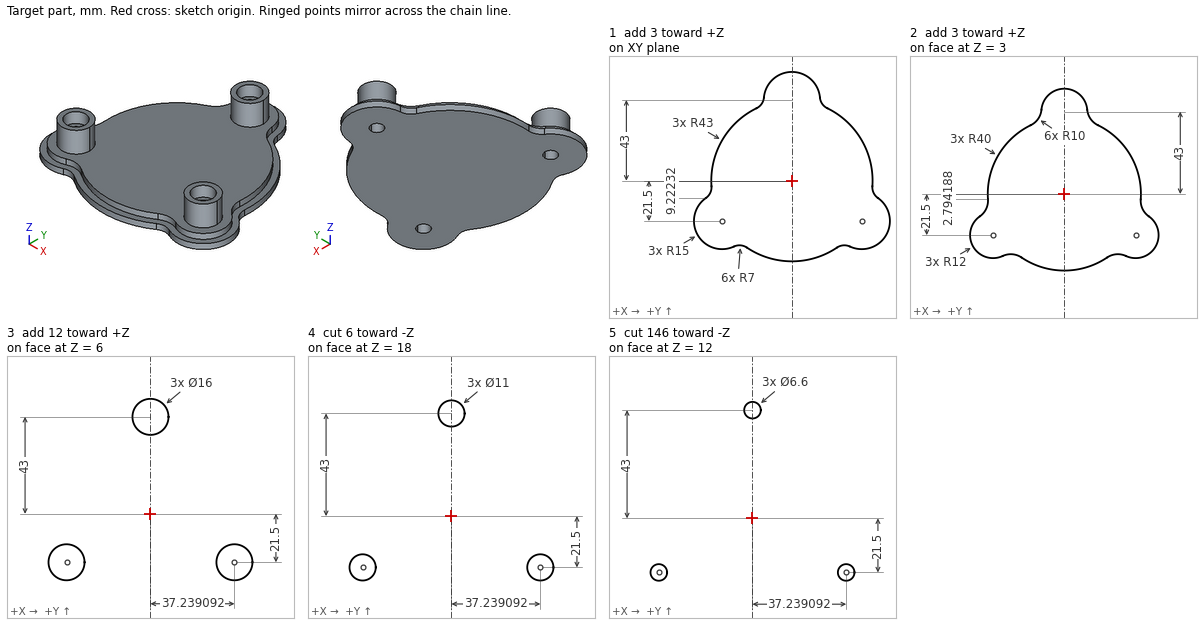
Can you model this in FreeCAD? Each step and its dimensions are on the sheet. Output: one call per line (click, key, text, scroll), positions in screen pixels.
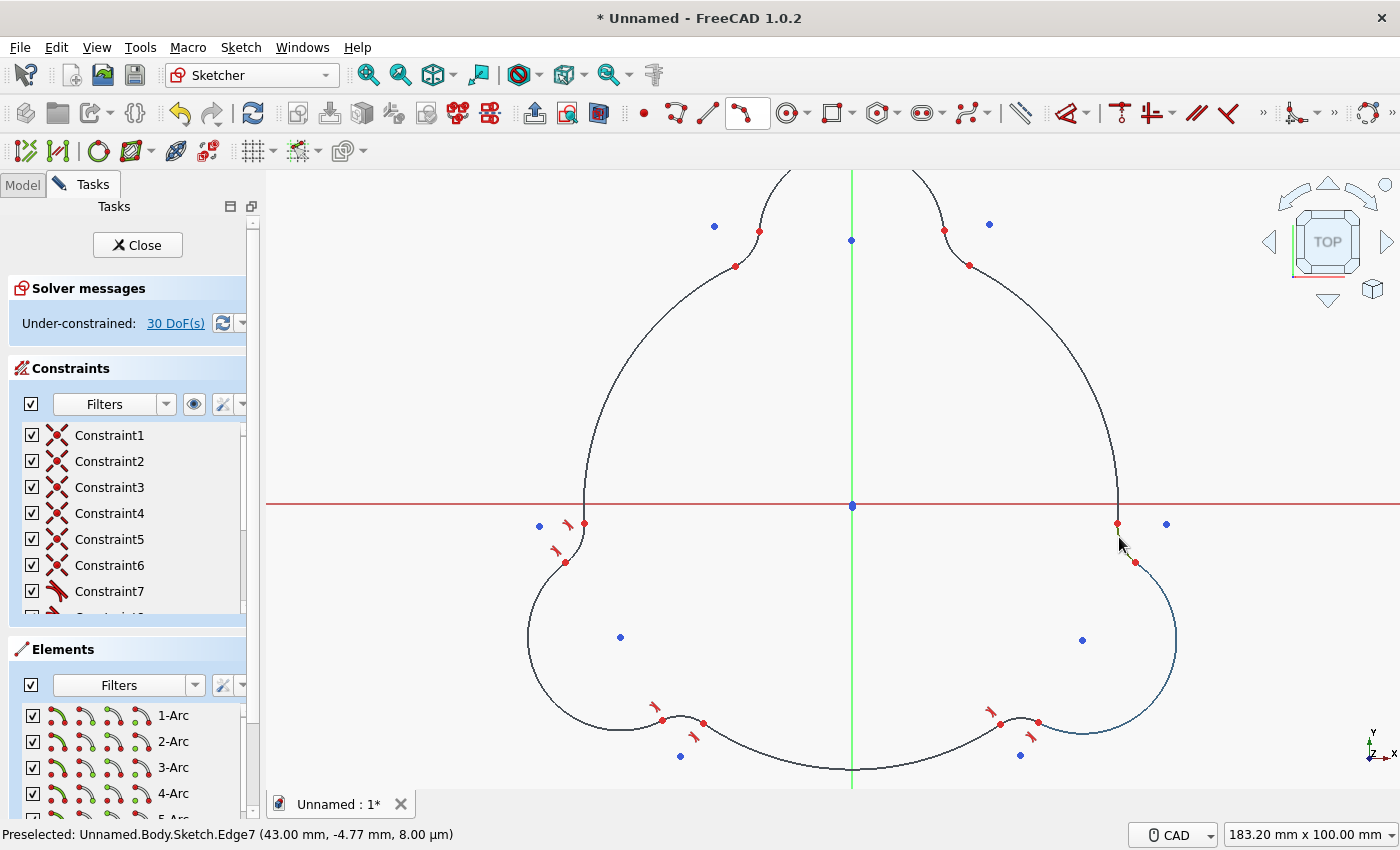
key(t)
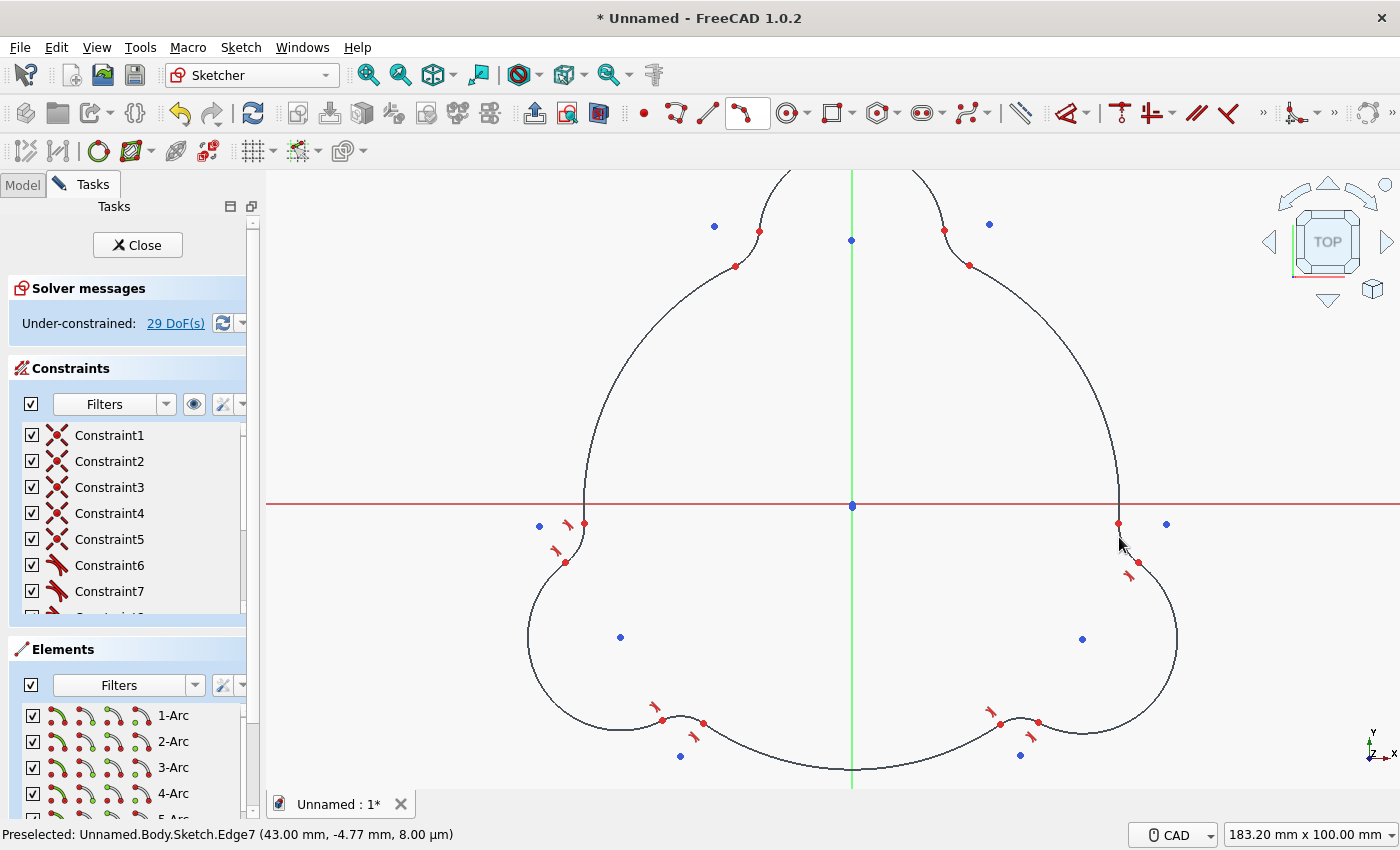
click(1121, 537)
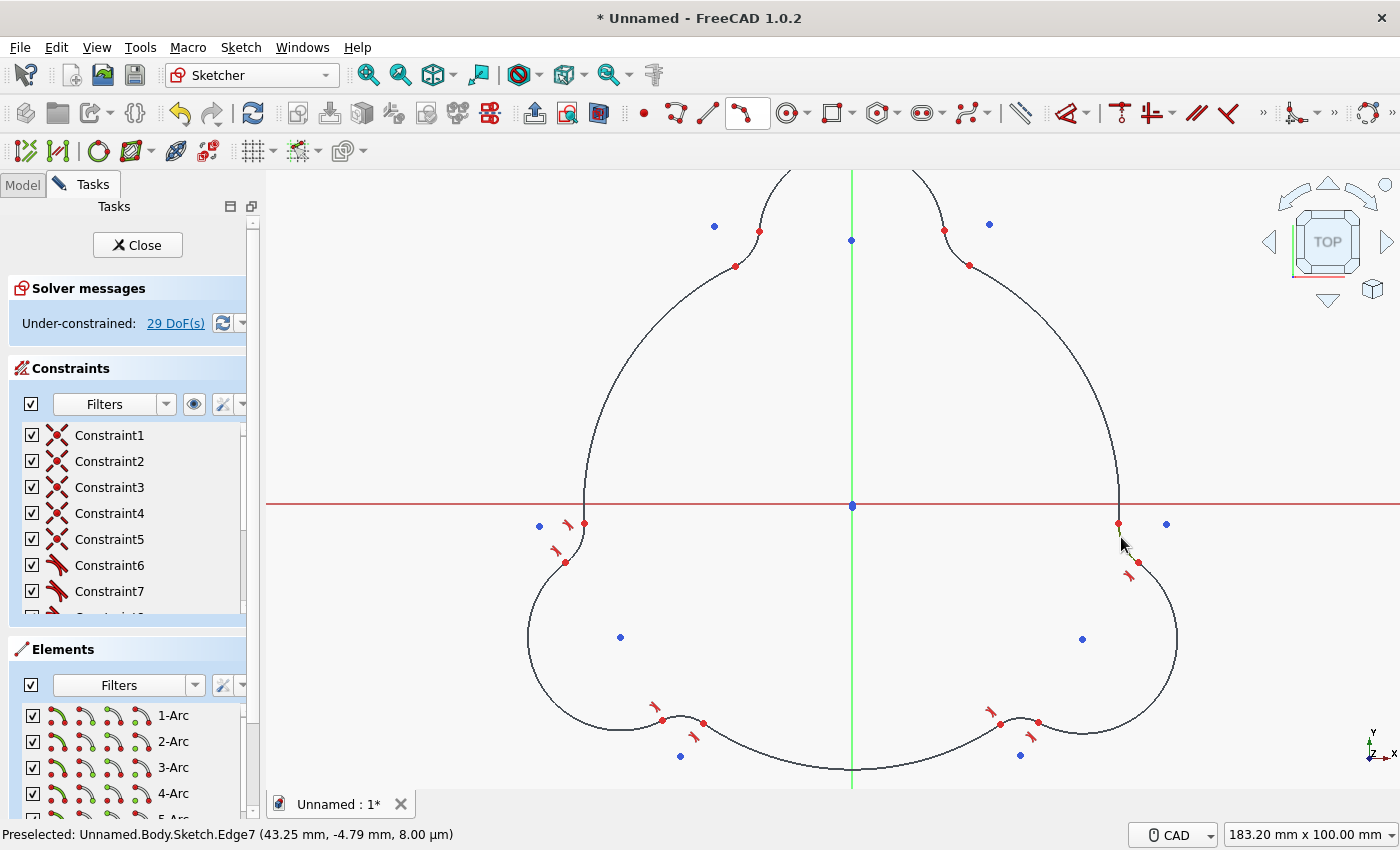
click(1108, 430)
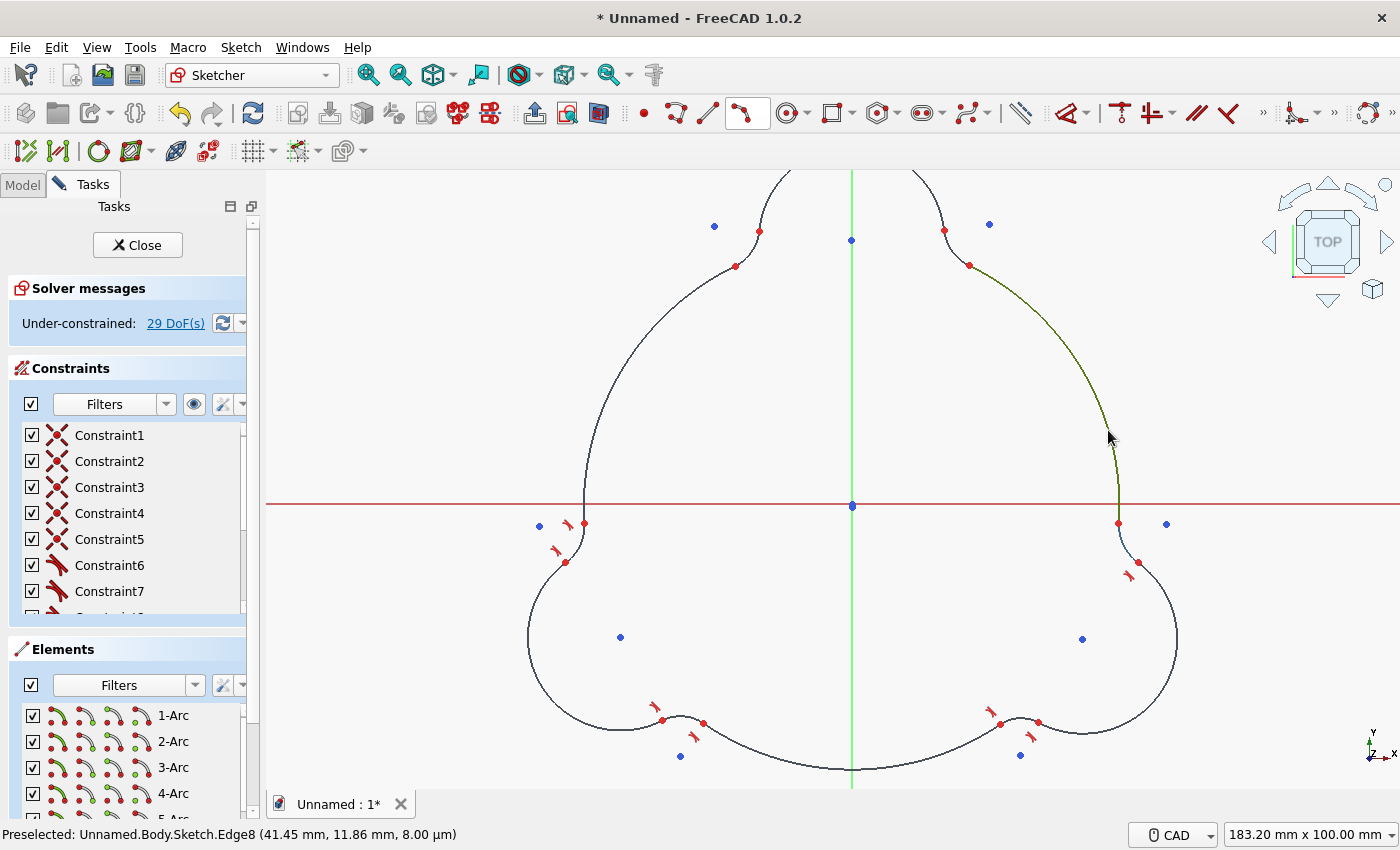
key(t)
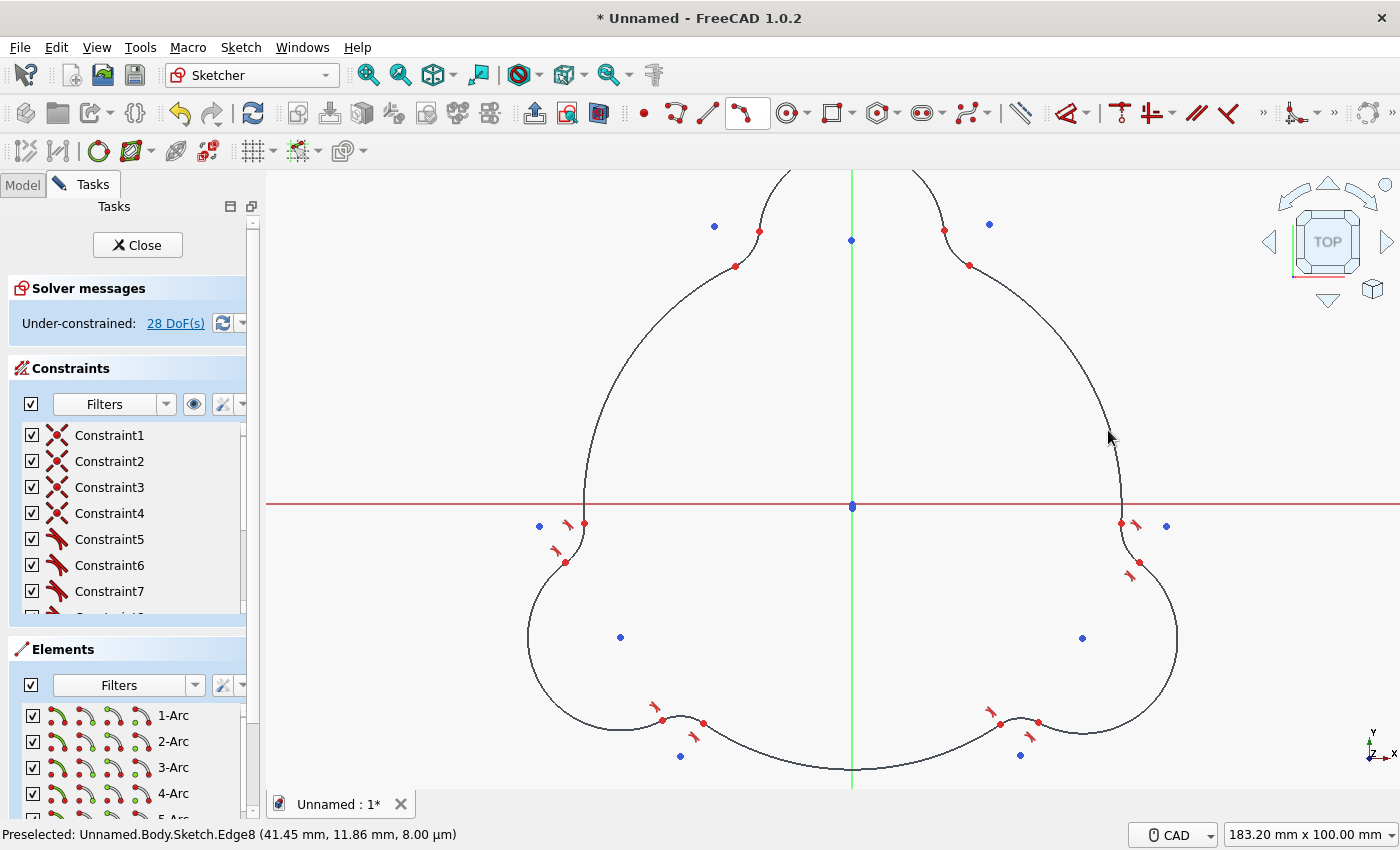
click(1110, 430)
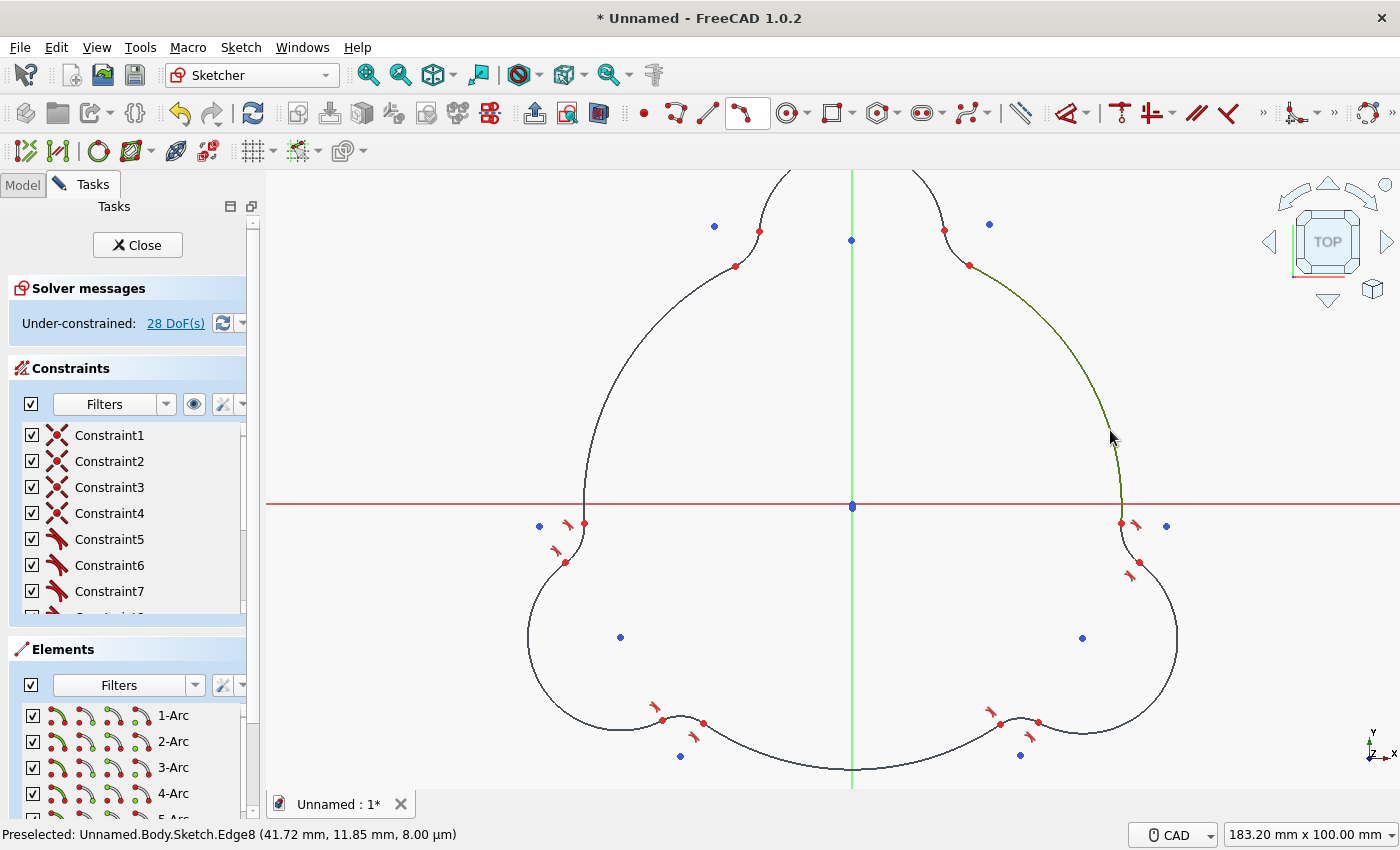
click(948, 243)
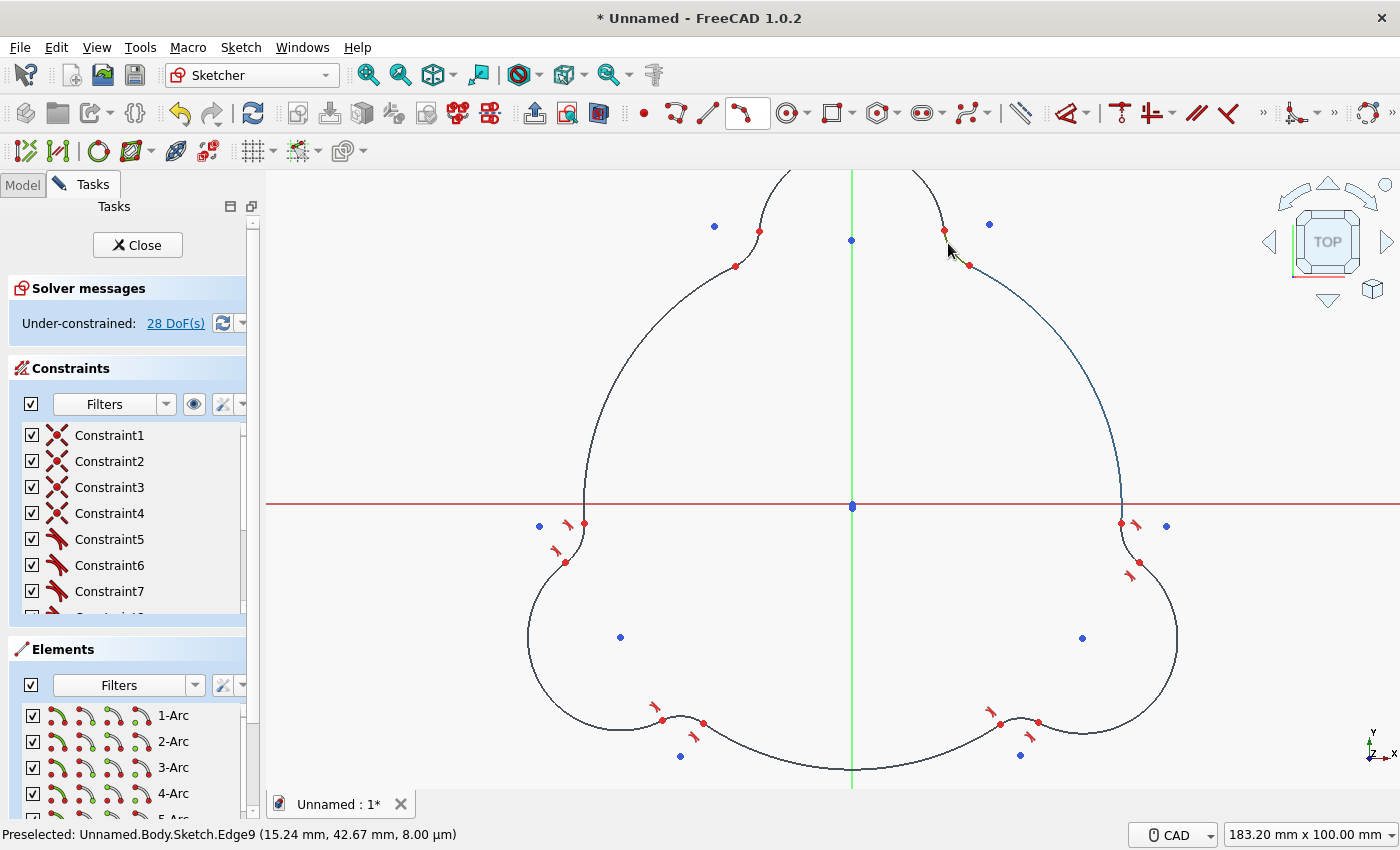
key(t)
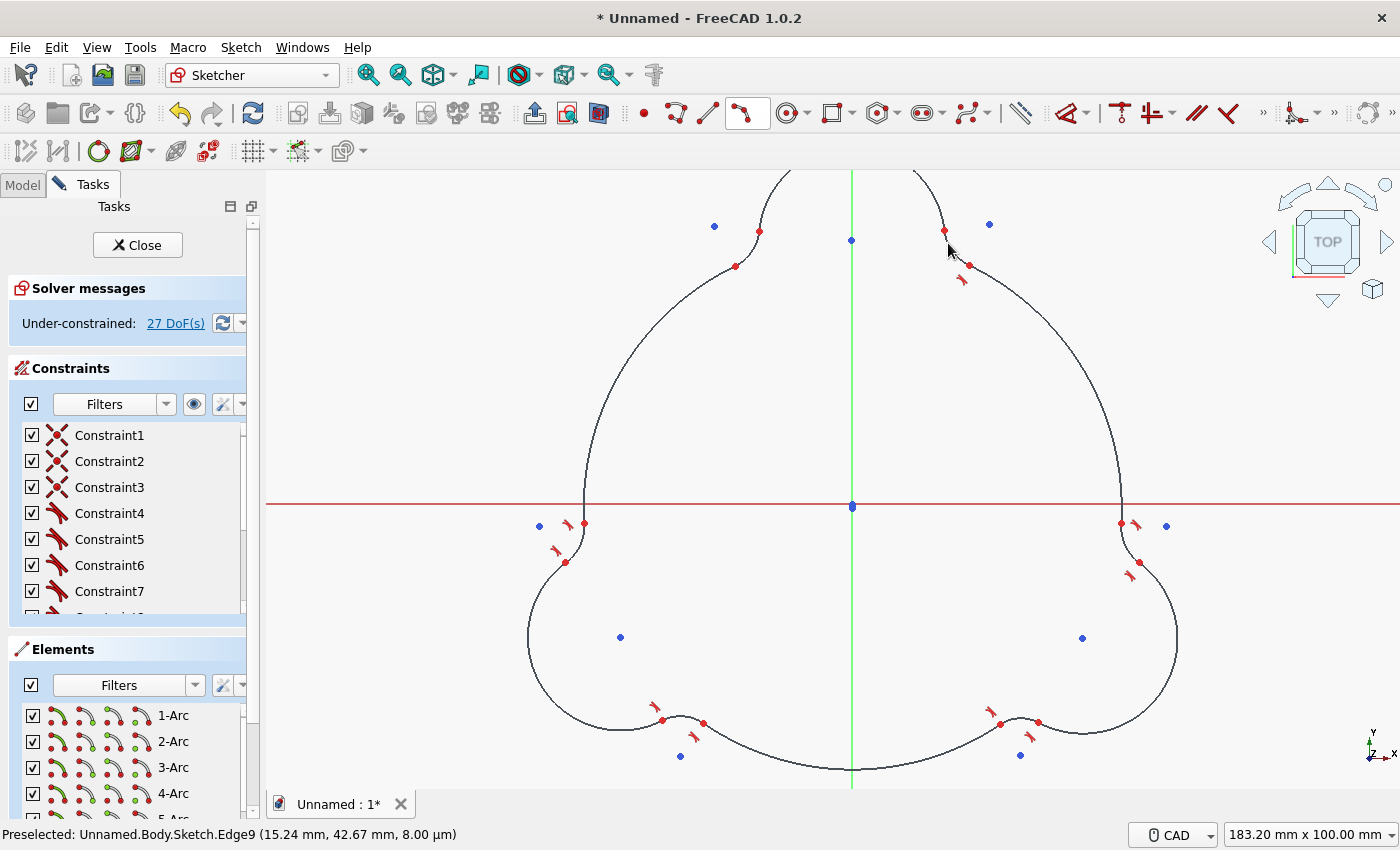
click(948, 243)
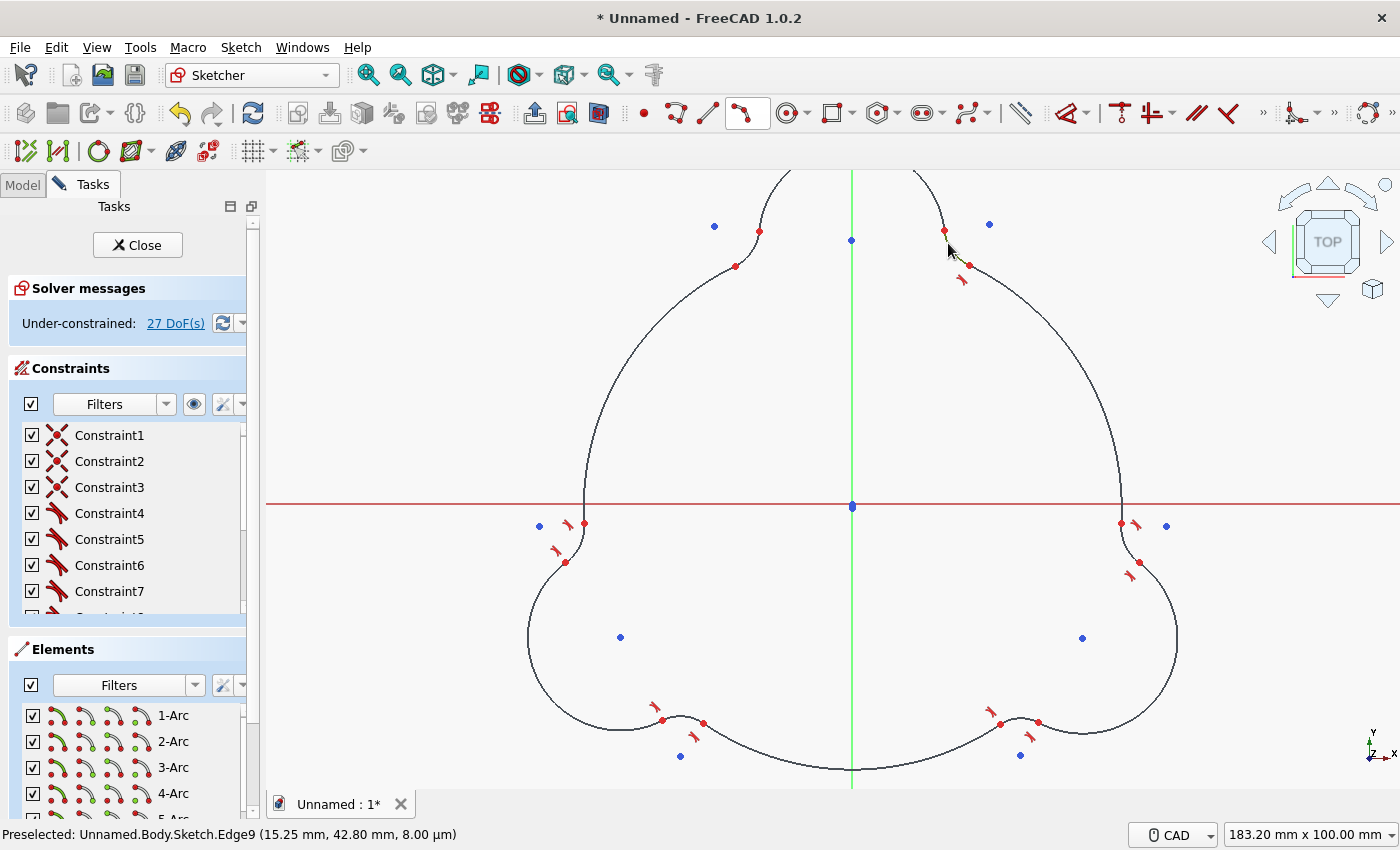
scroll(586, 524, down, 2)